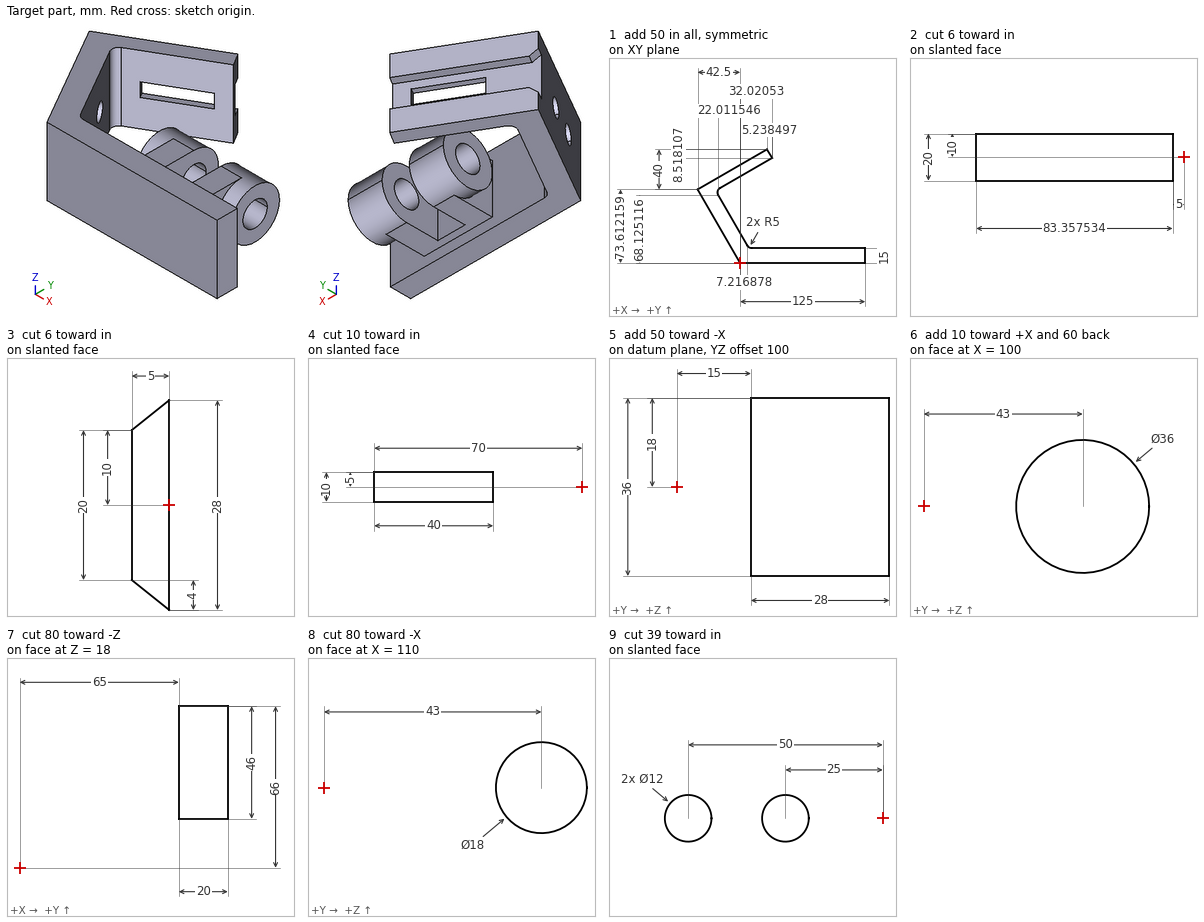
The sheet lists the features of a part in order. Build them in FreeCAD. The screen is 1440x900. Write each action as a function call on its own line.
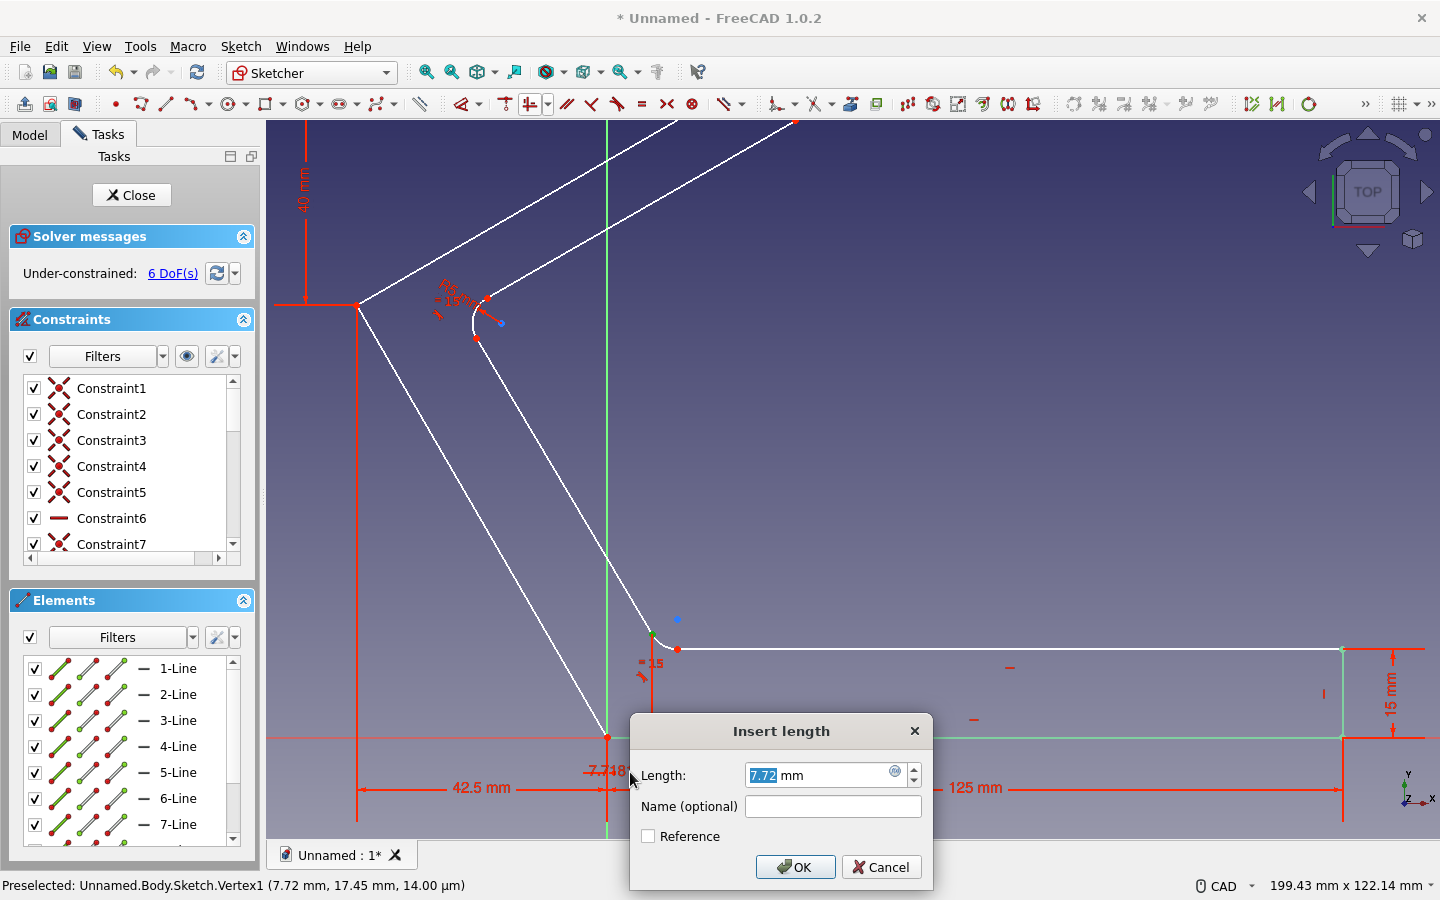
text(7.216878)
key(Return)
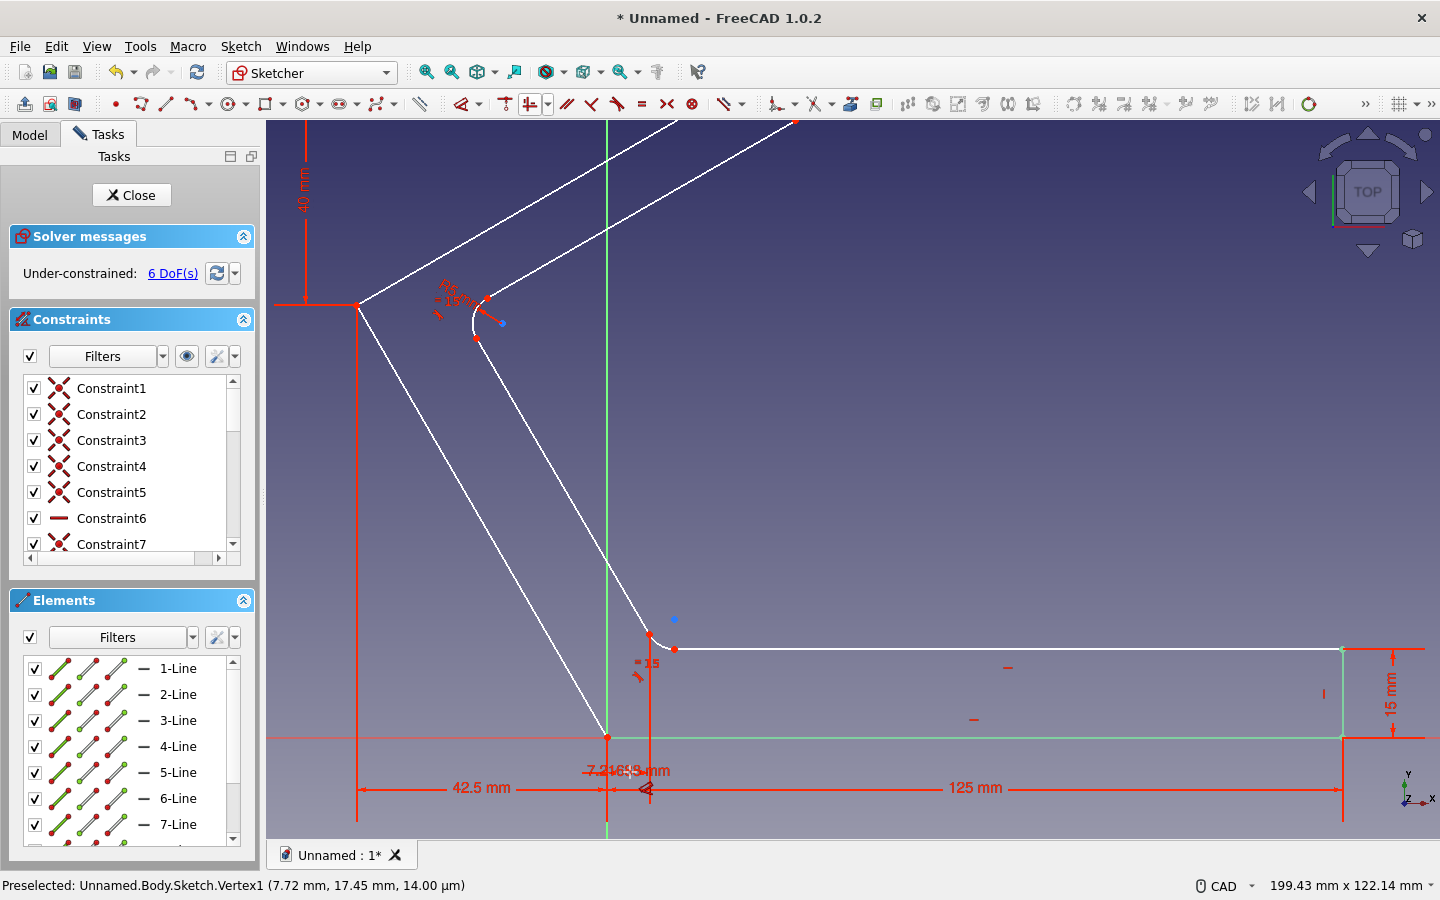
scroll(652, 635, down, 2)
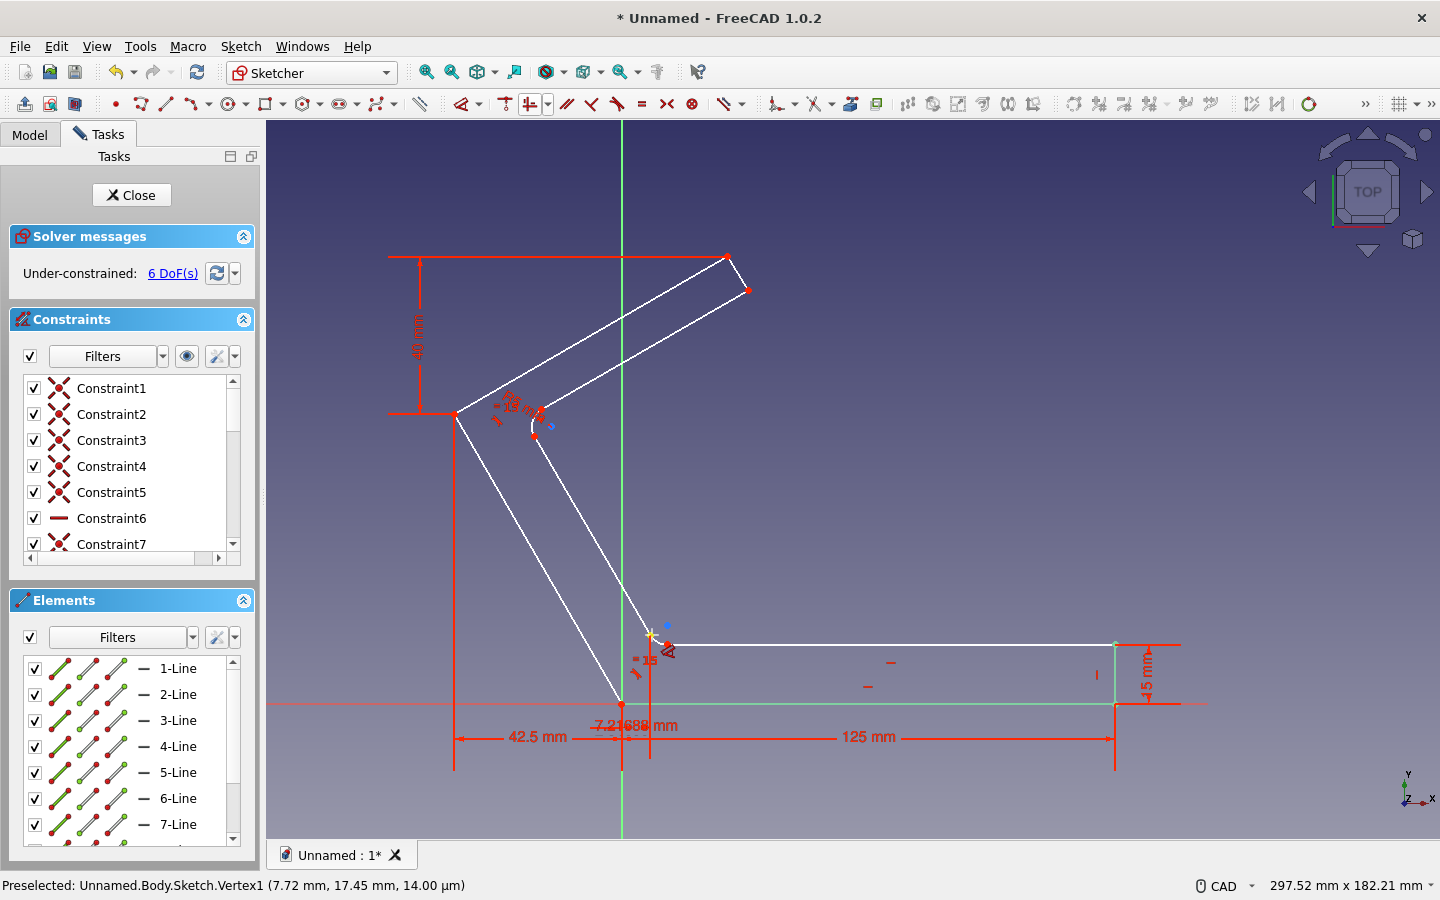
click(748, 291)
click(714, 738)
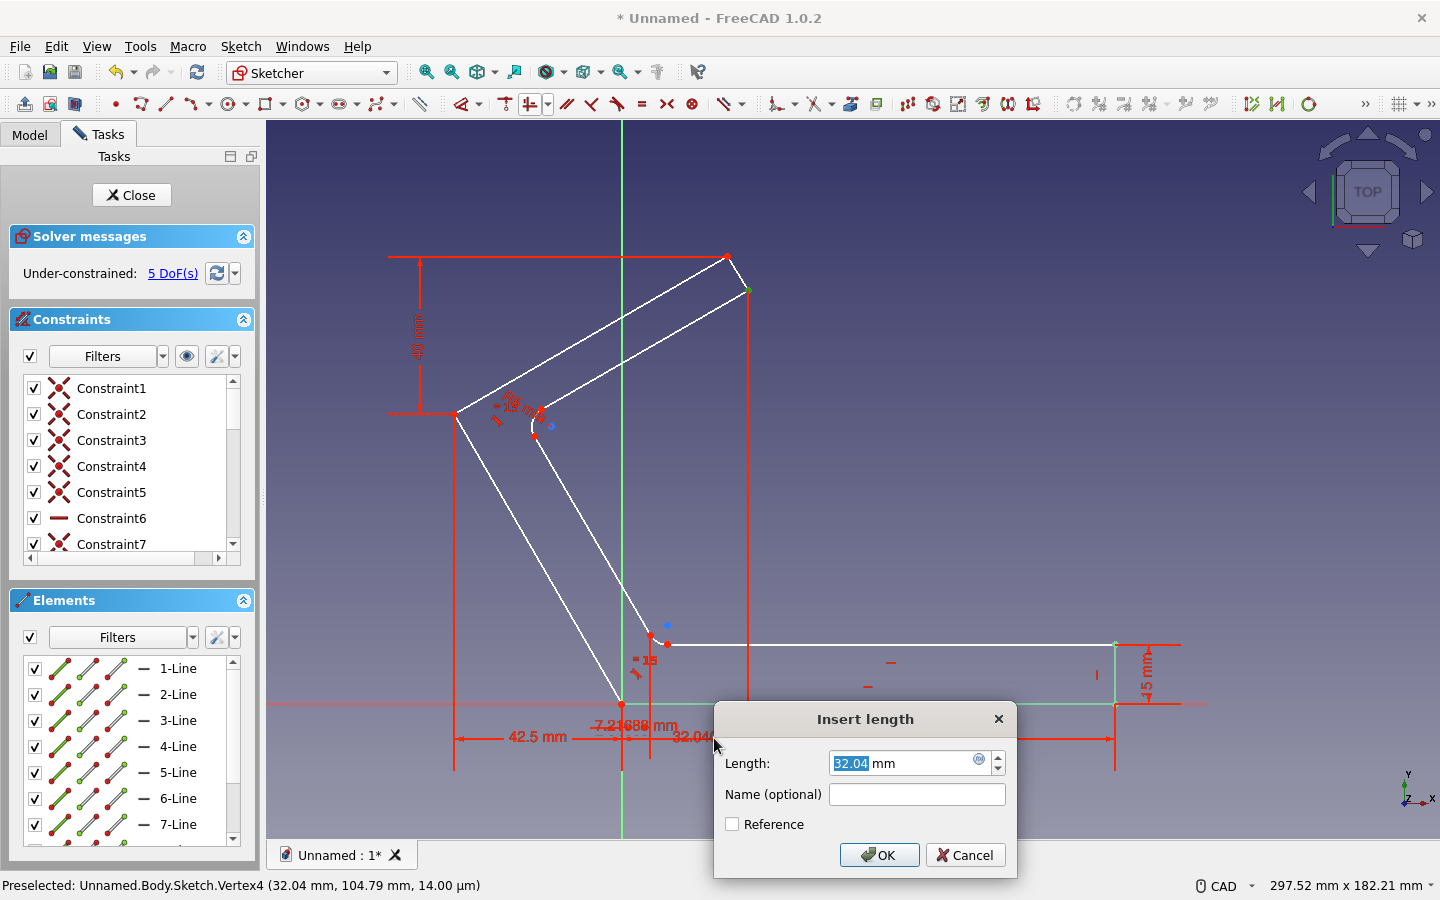
text(32.02053)
key(Return)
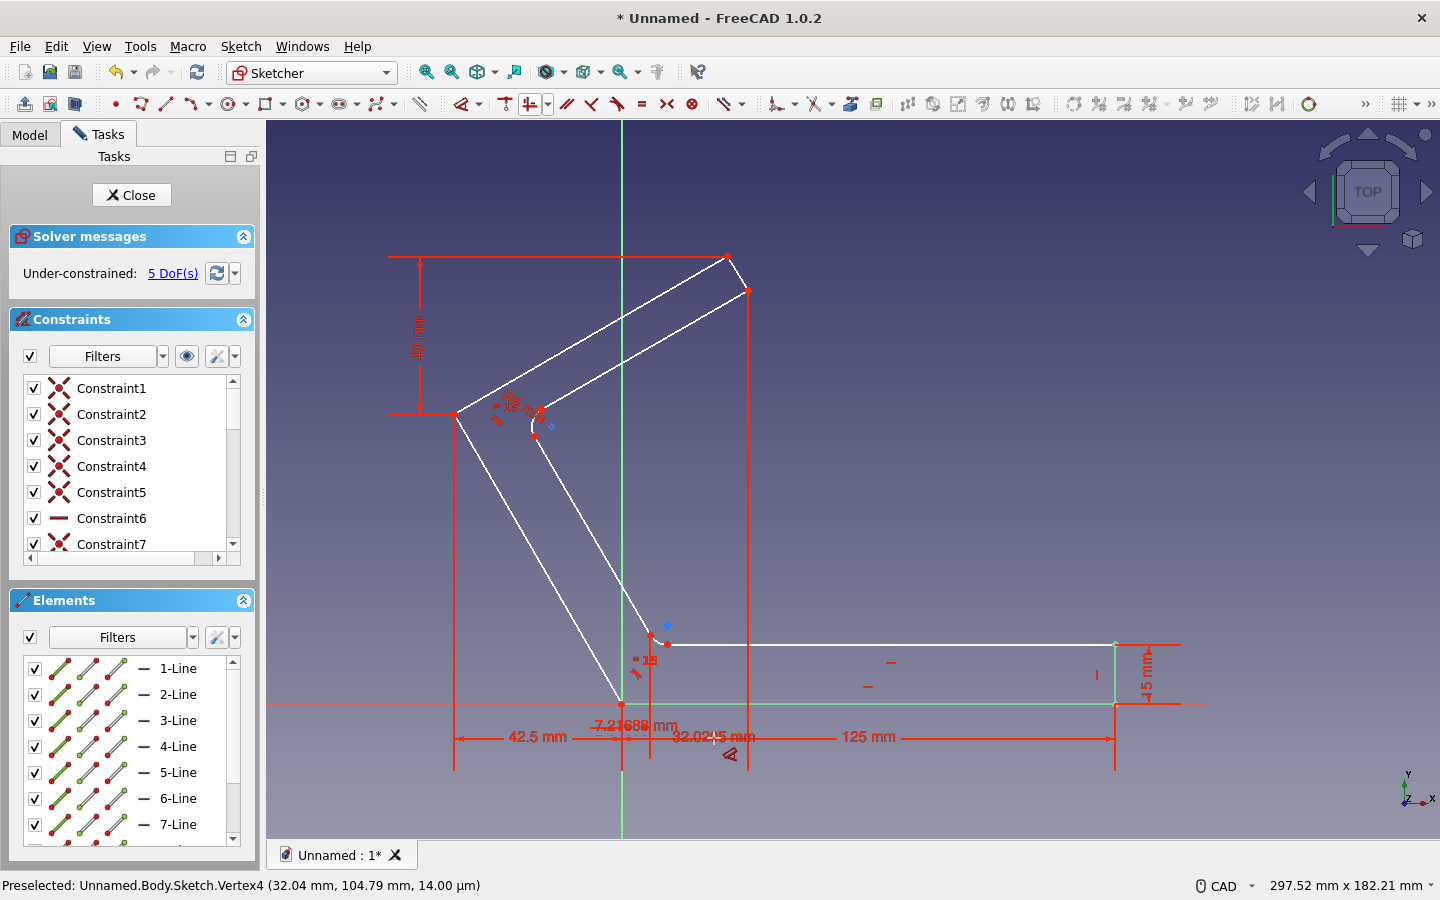
scroll(742, 280, up, 4)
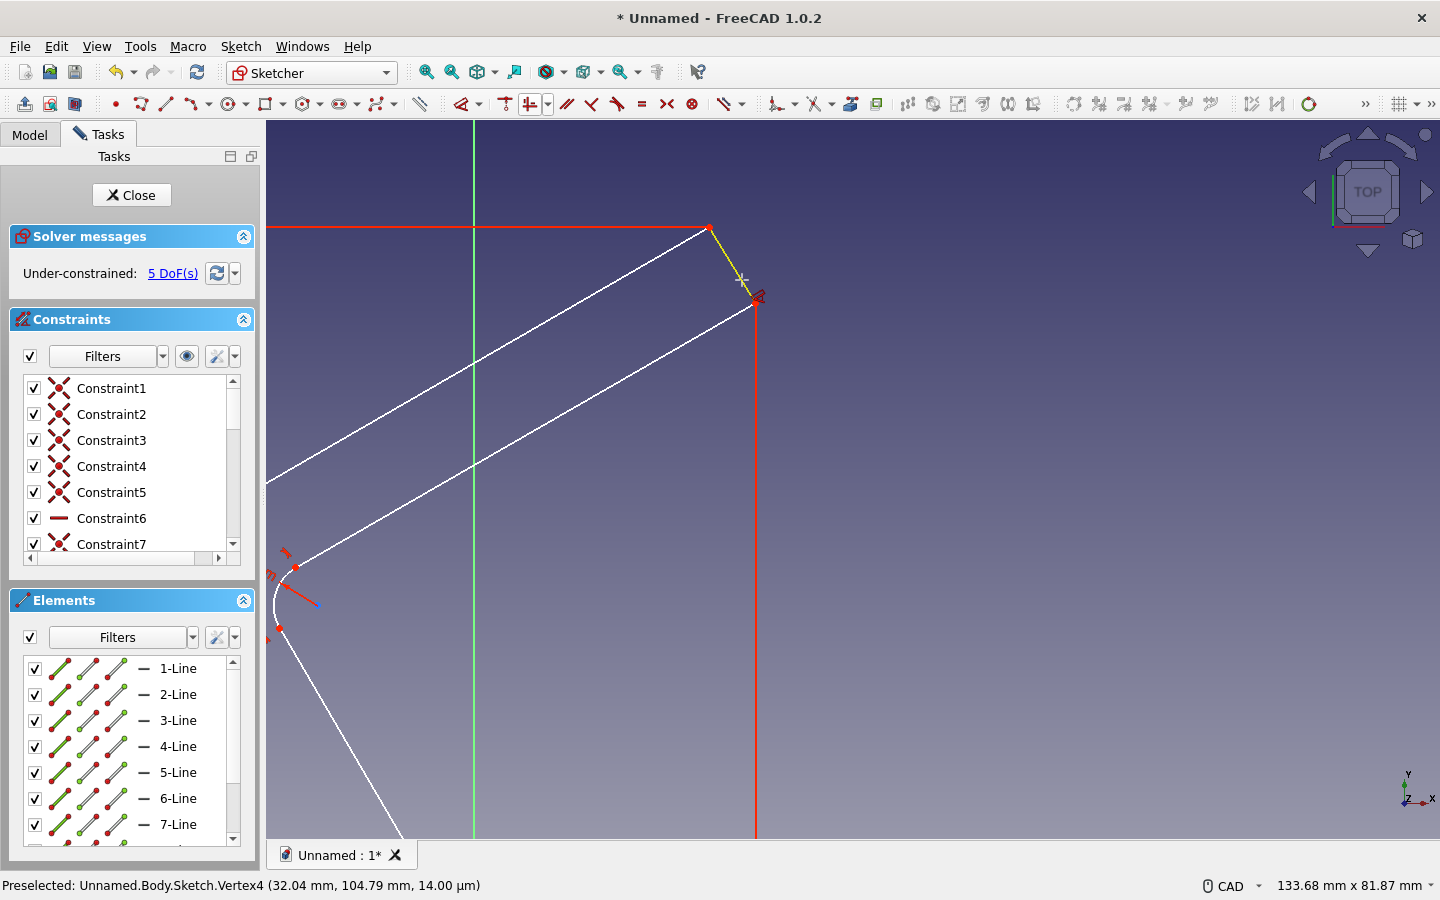
click(742, 280)
click(732, 193)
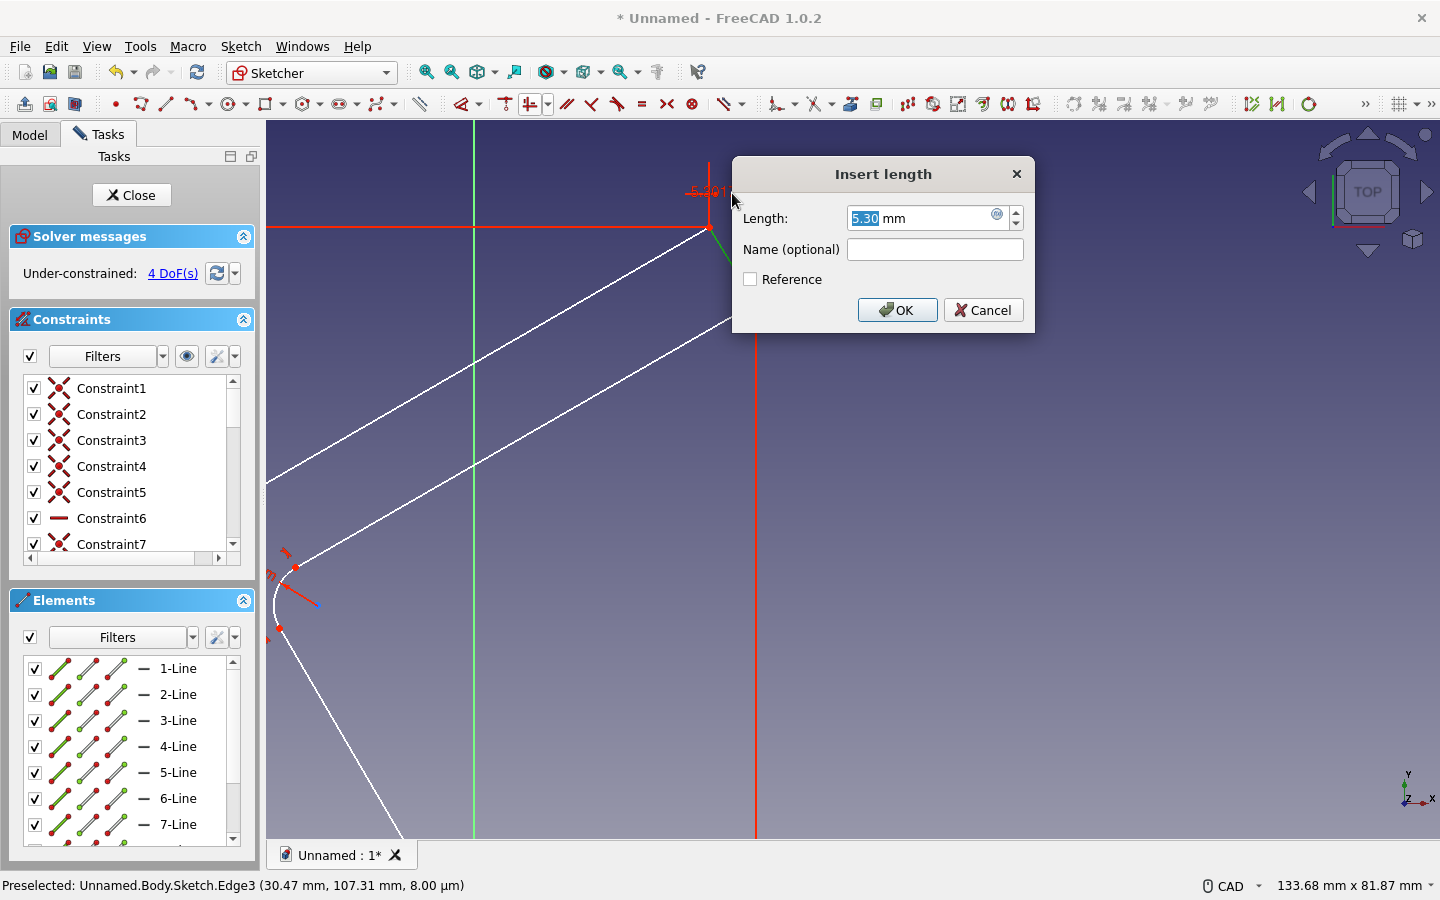
text(5.238497)
key(Return)